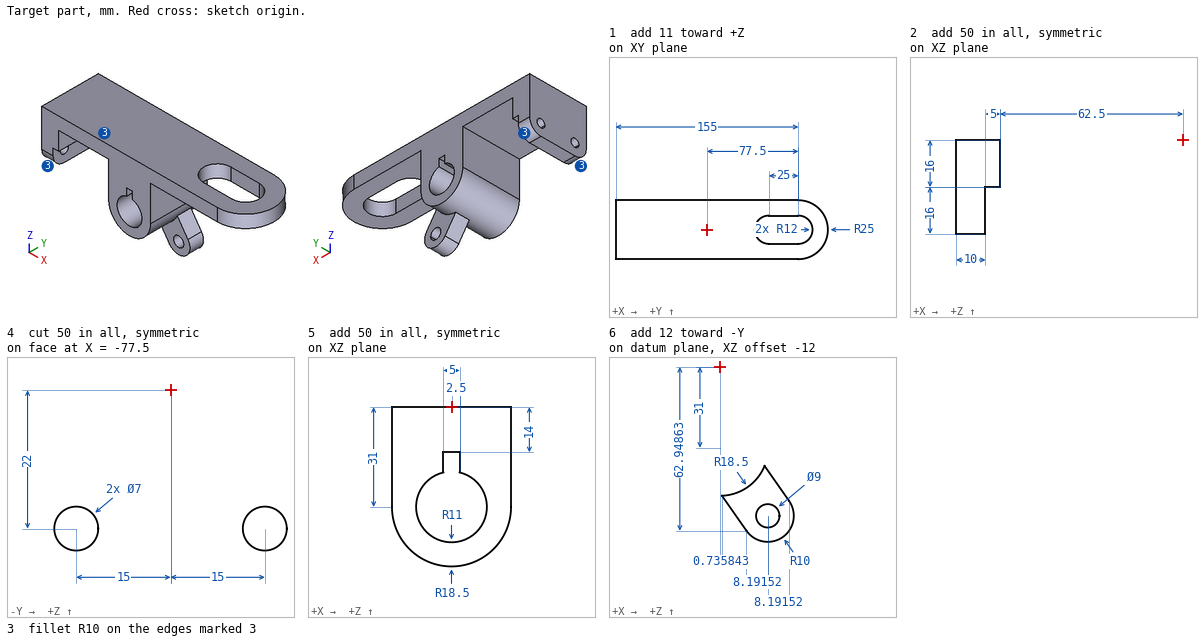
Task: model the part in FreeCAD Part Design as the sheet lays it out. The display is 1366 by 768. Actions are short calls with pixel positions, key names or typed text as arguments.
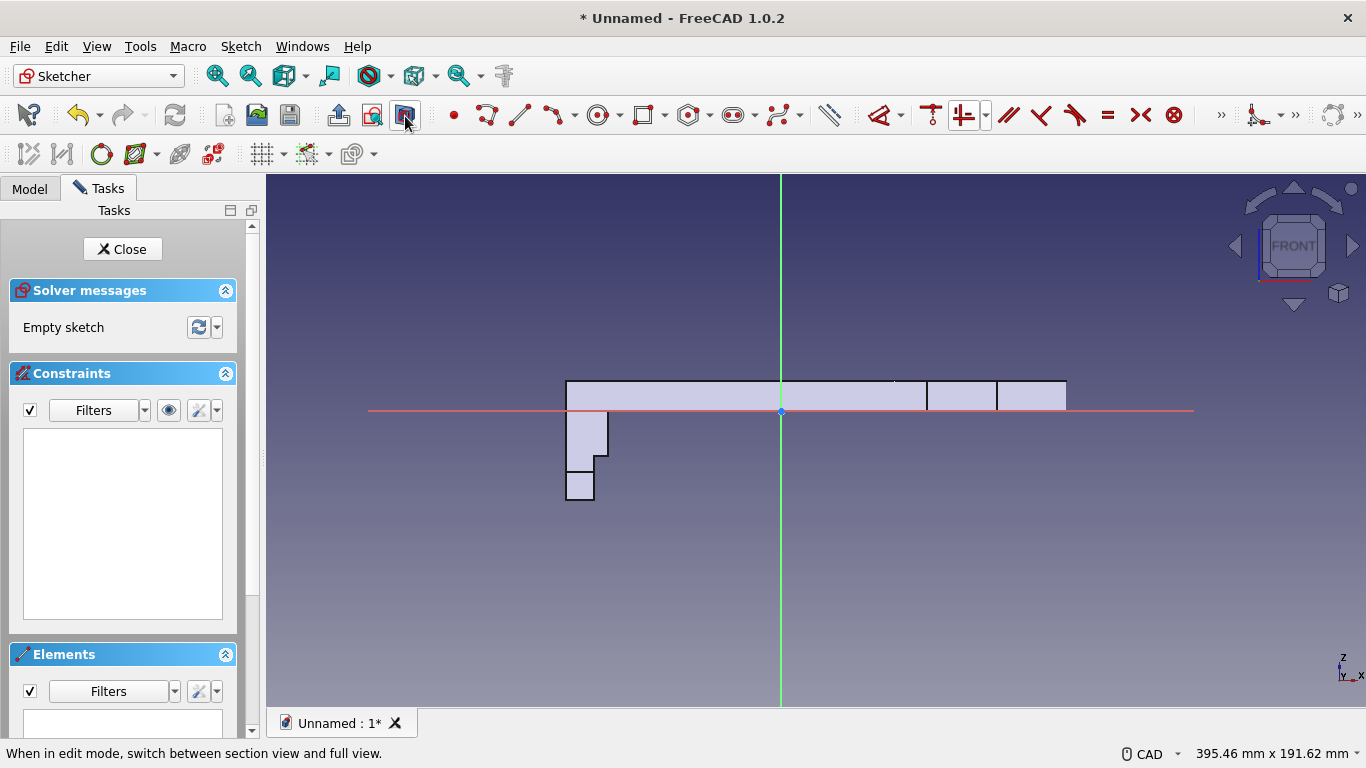
scroll(809, 512, up, 4)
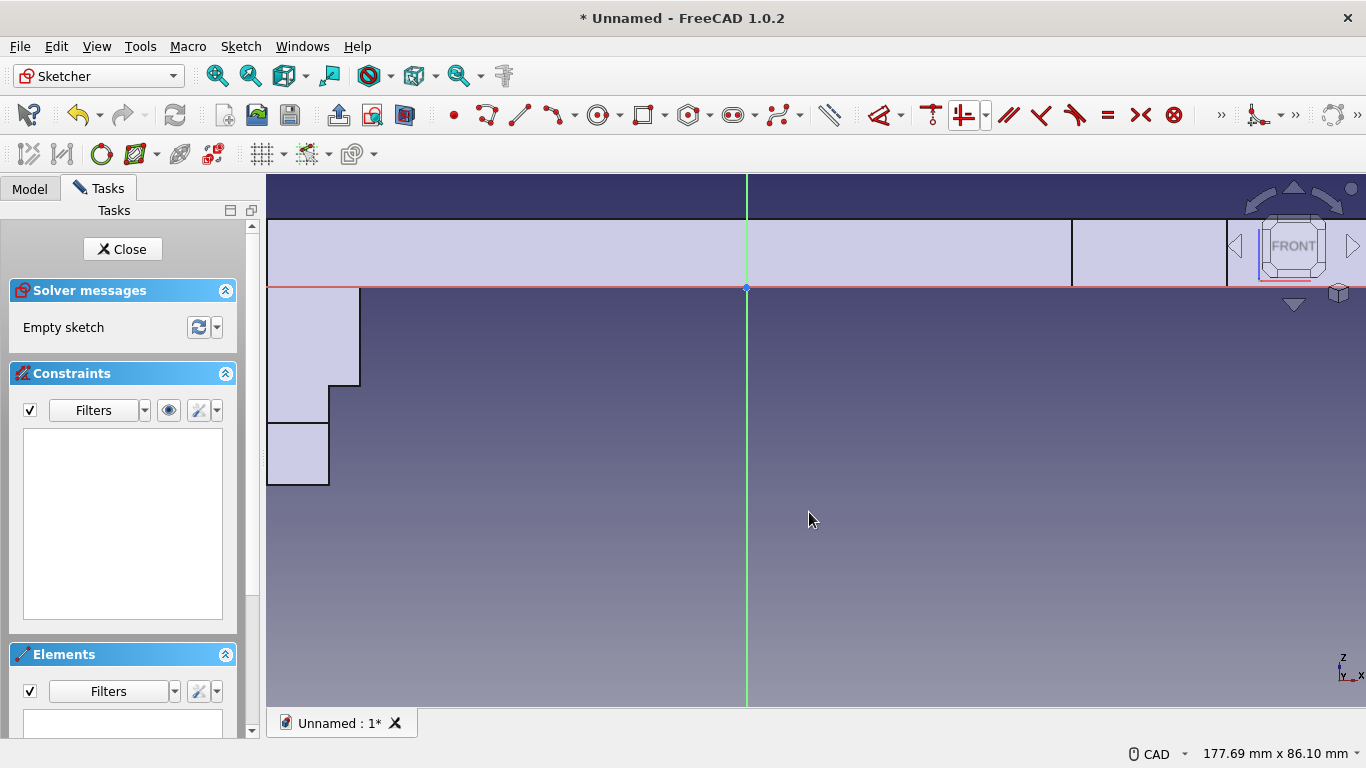
click(487, 116)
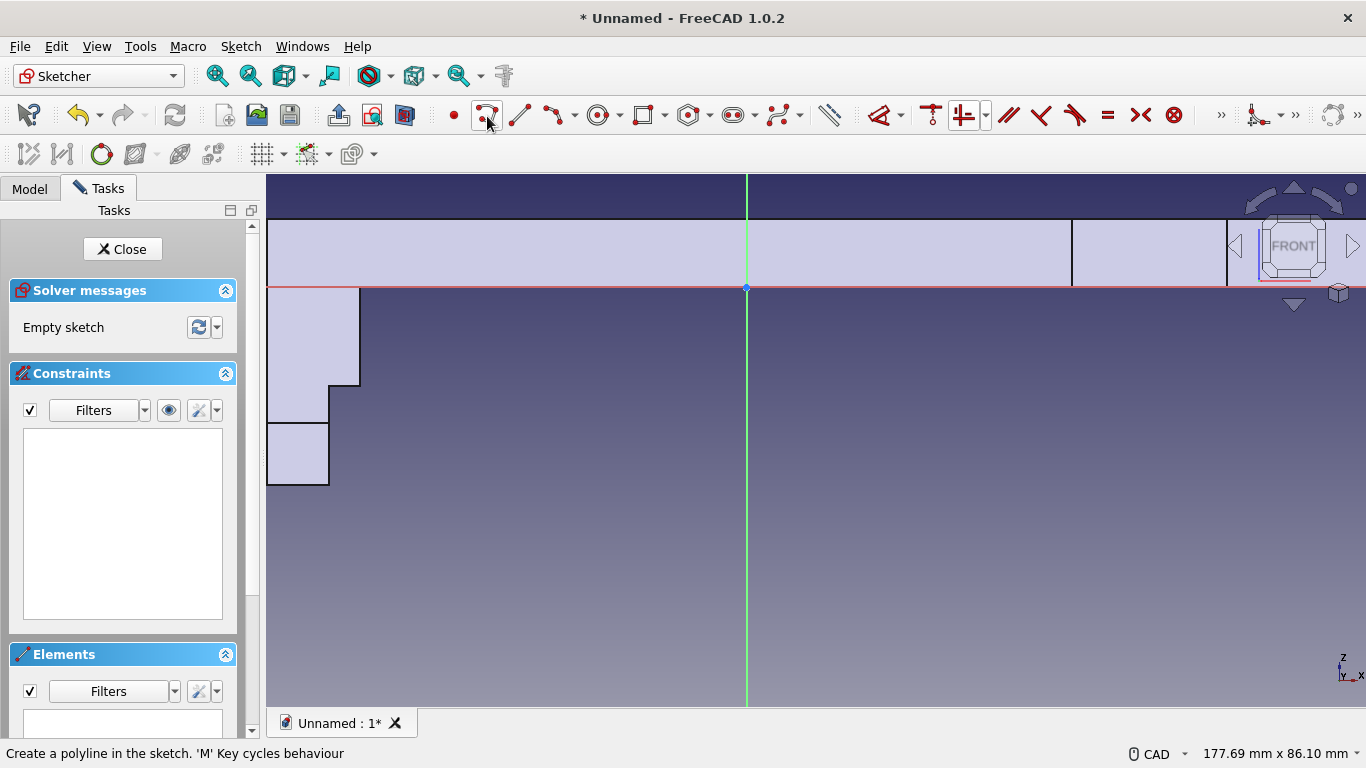
click(632, 479)
click(632, 287)
click(861, 296)
click(861, 479)
right_click(861, 479)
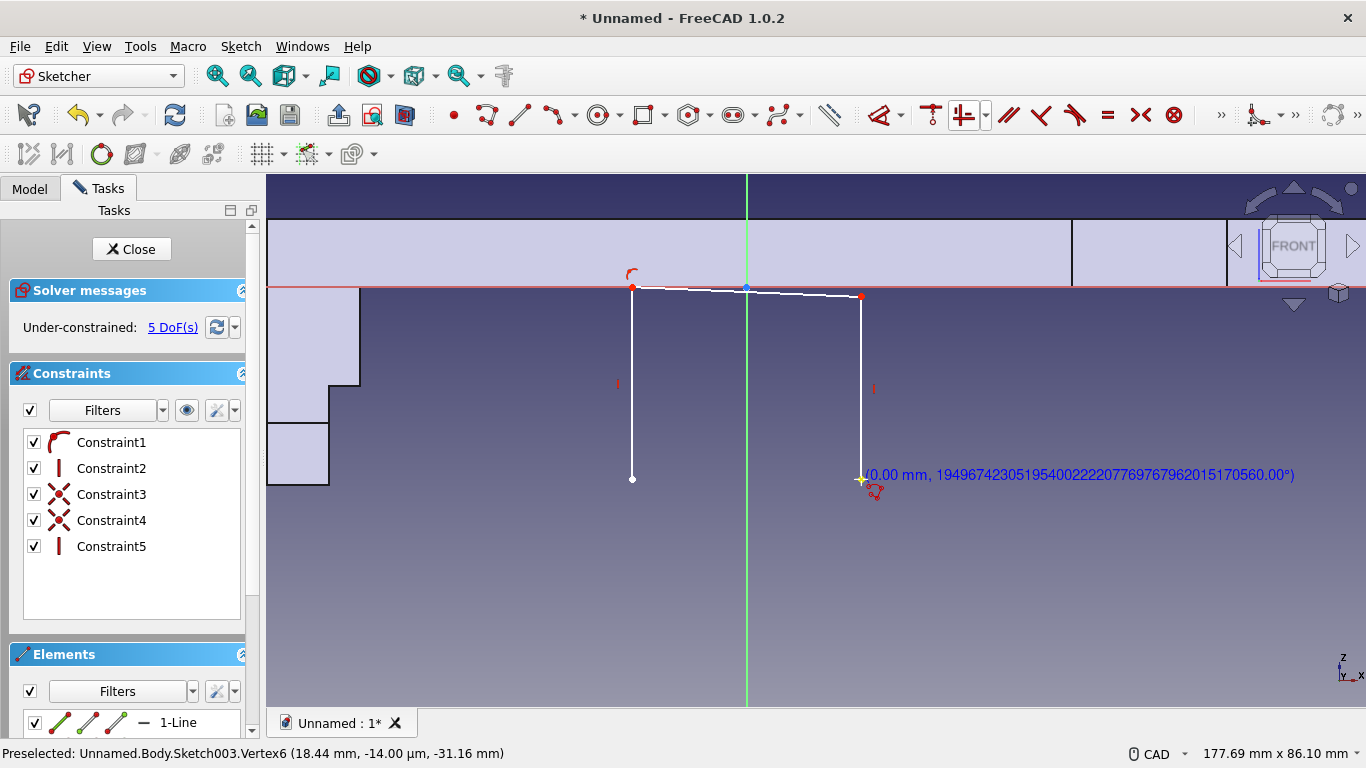
click(552, 116)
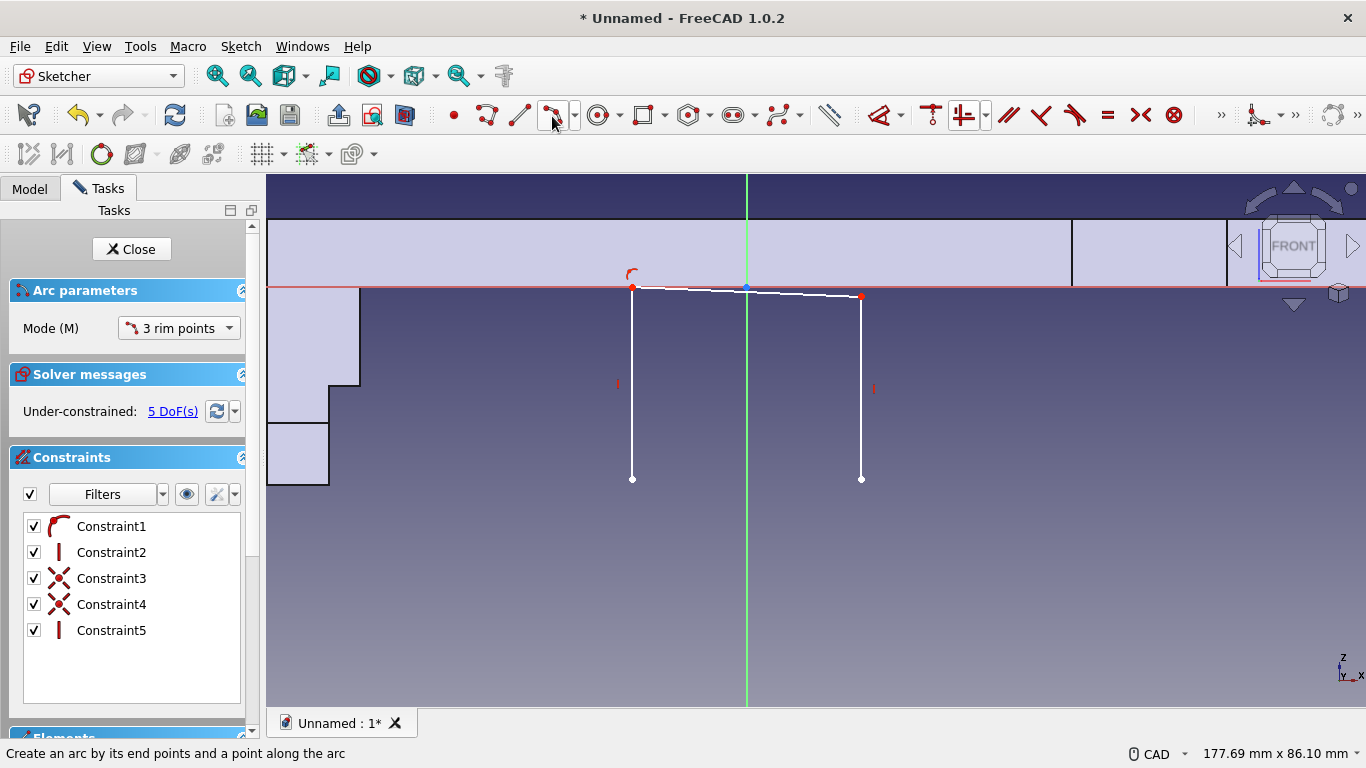
click(861, 480)
click(632, 480)
click(711, 588)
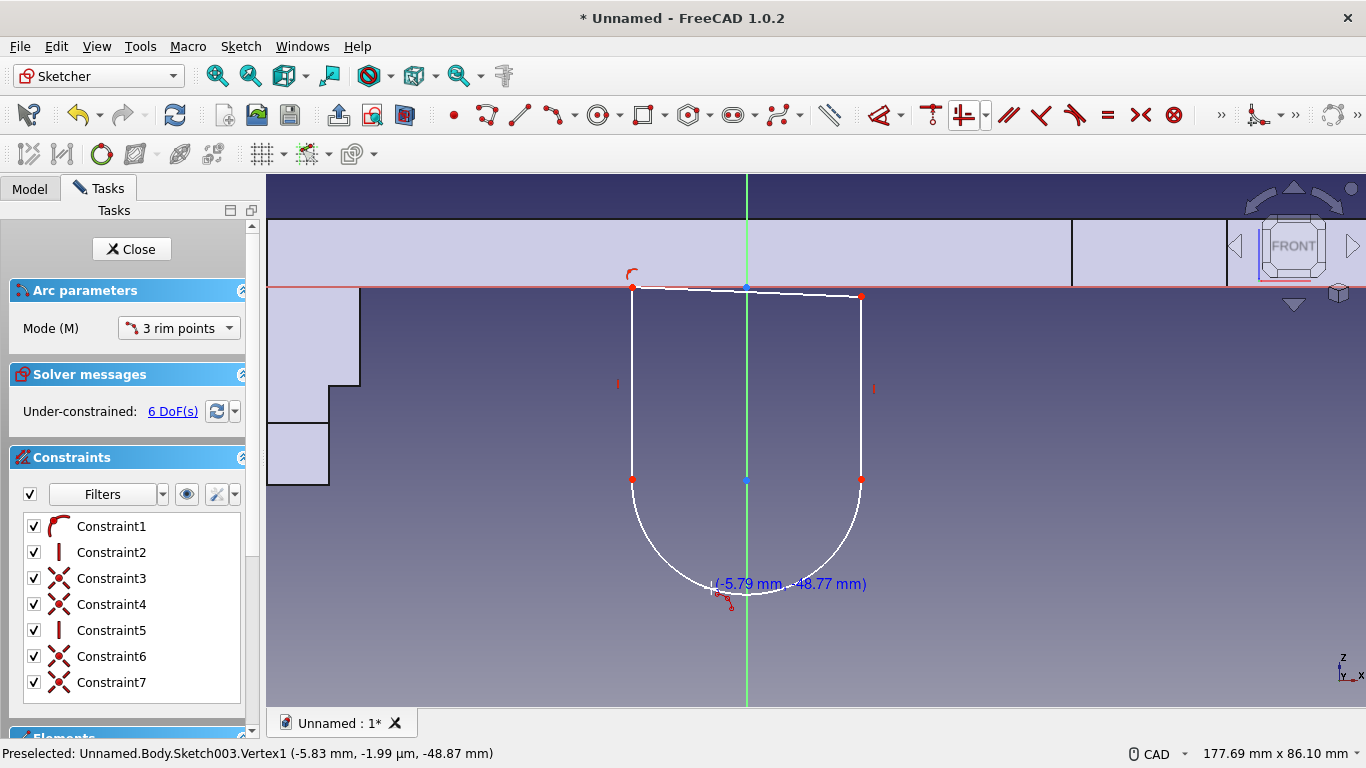
key(g)
key(m)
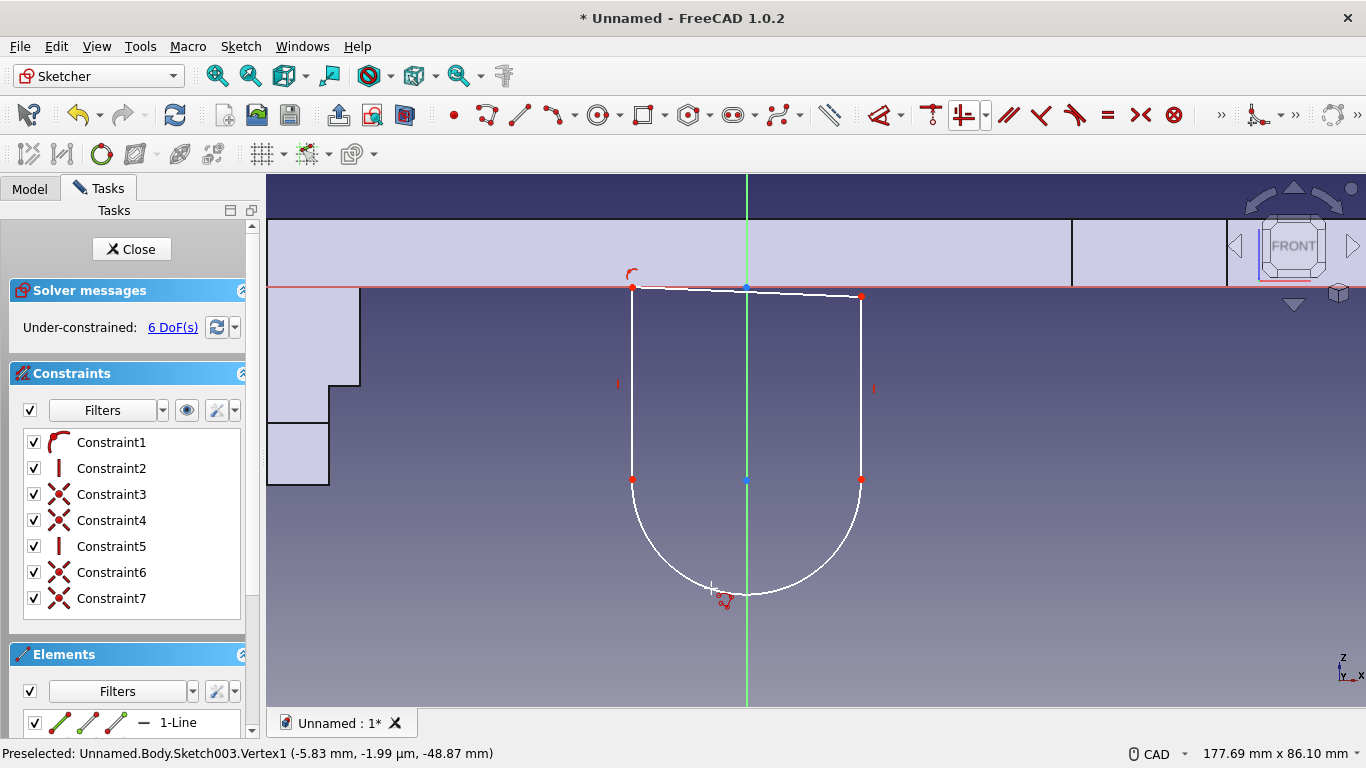
click(762, 413)
click(762, 374)
click(731, 374)
click(731, 413)
right_click(731, 413)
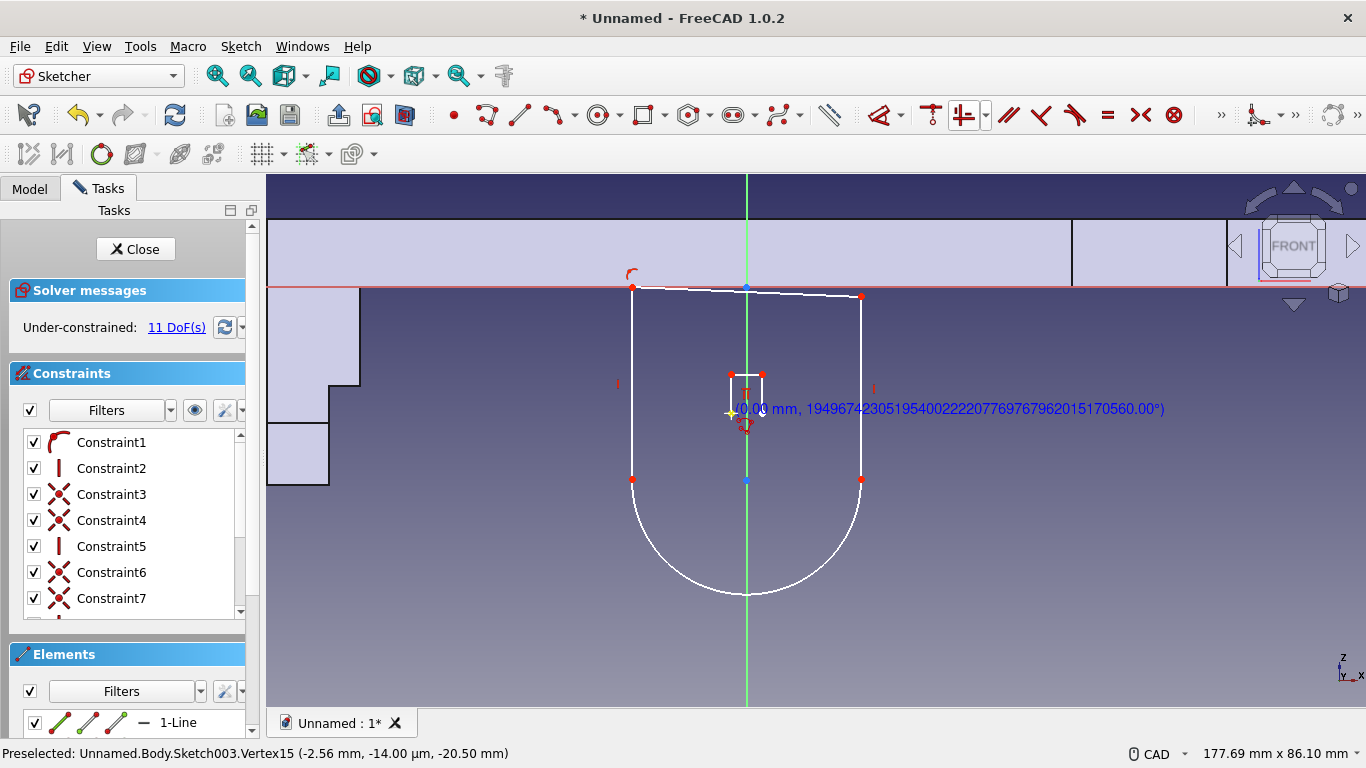
click(552, 116)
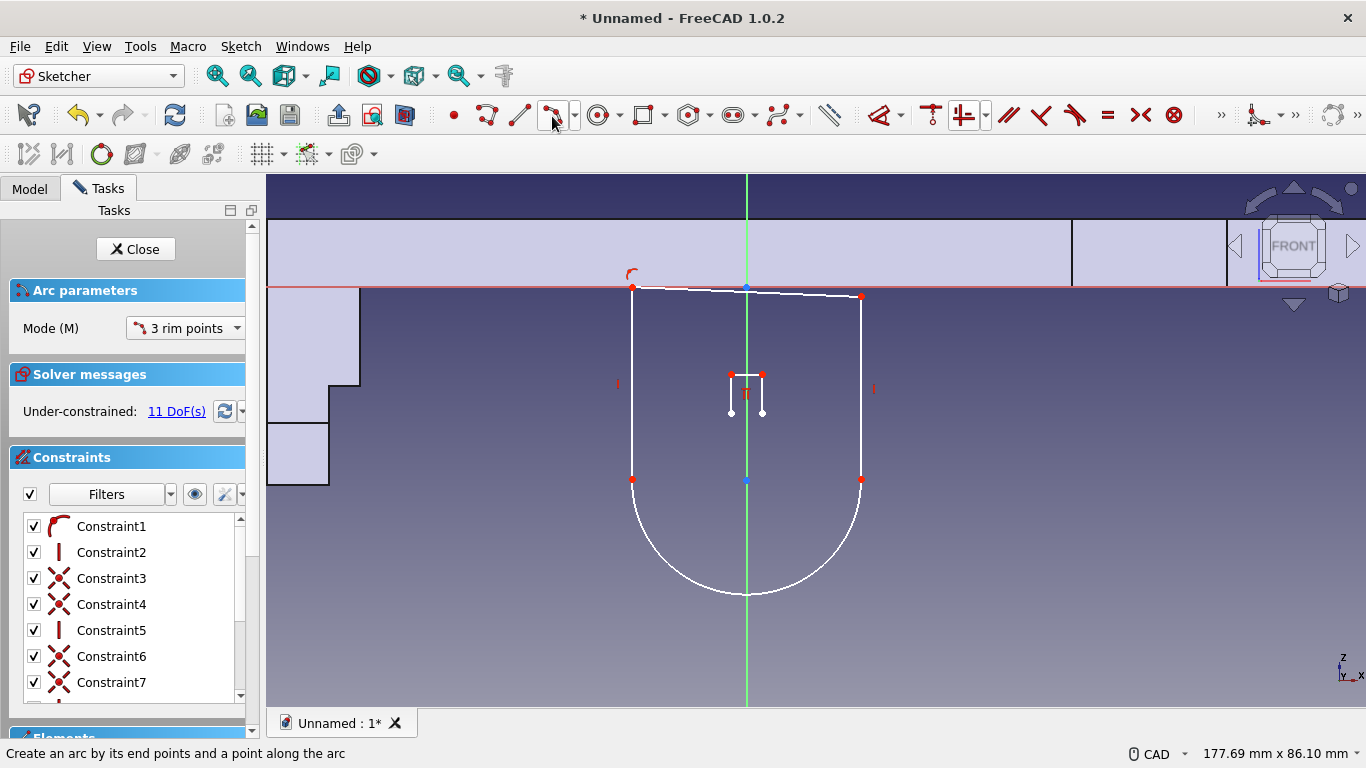
click(731, 414)
click(762, 414)
click(709, 536)
key(Escape)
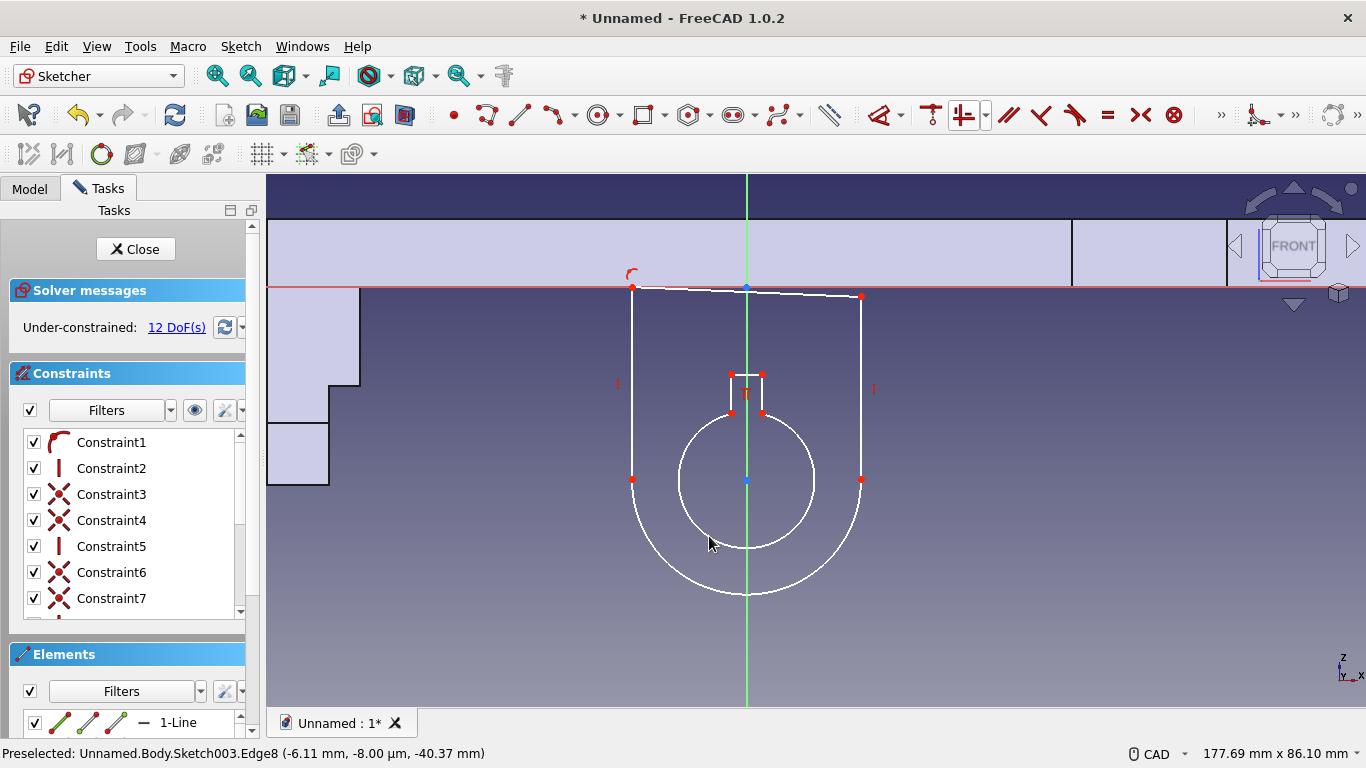
click(632, 422)